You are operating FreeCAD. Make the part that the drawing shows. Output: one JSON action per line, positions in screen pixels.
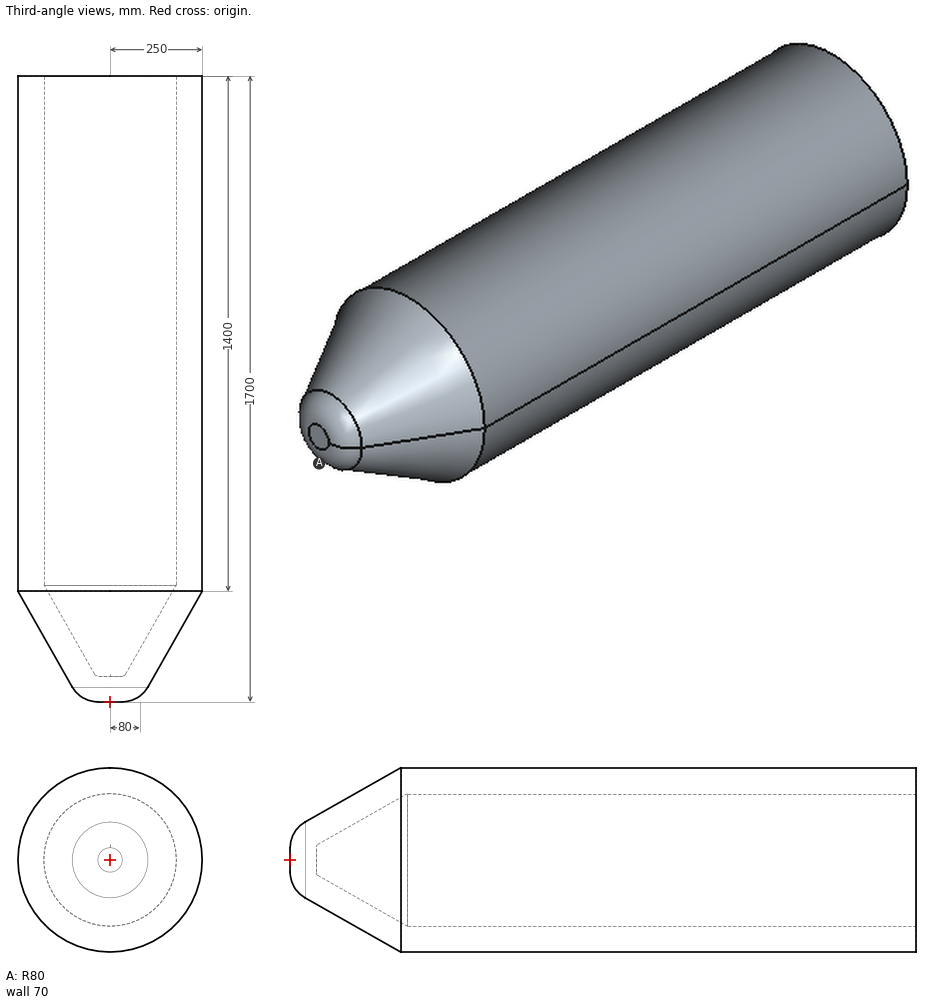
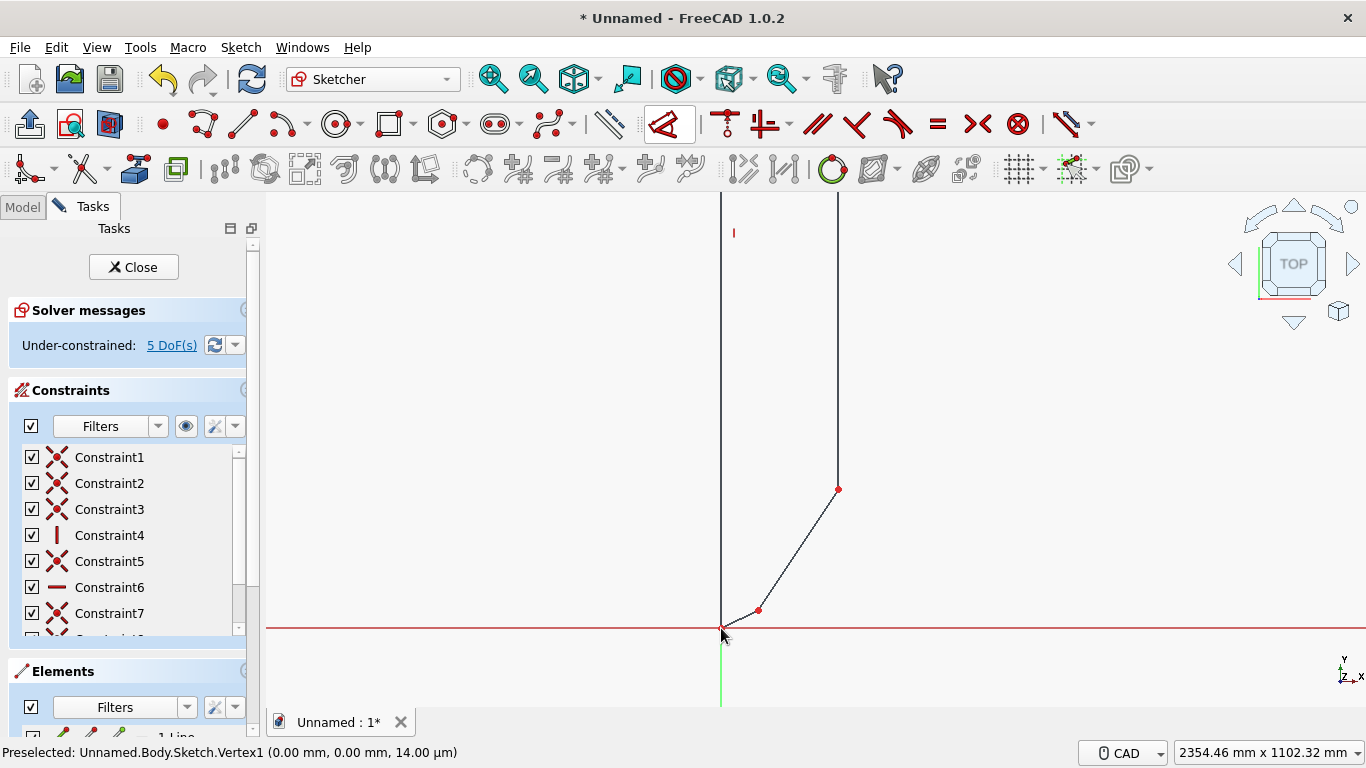
{"action": "left_click", "coordinate": [747, 616]}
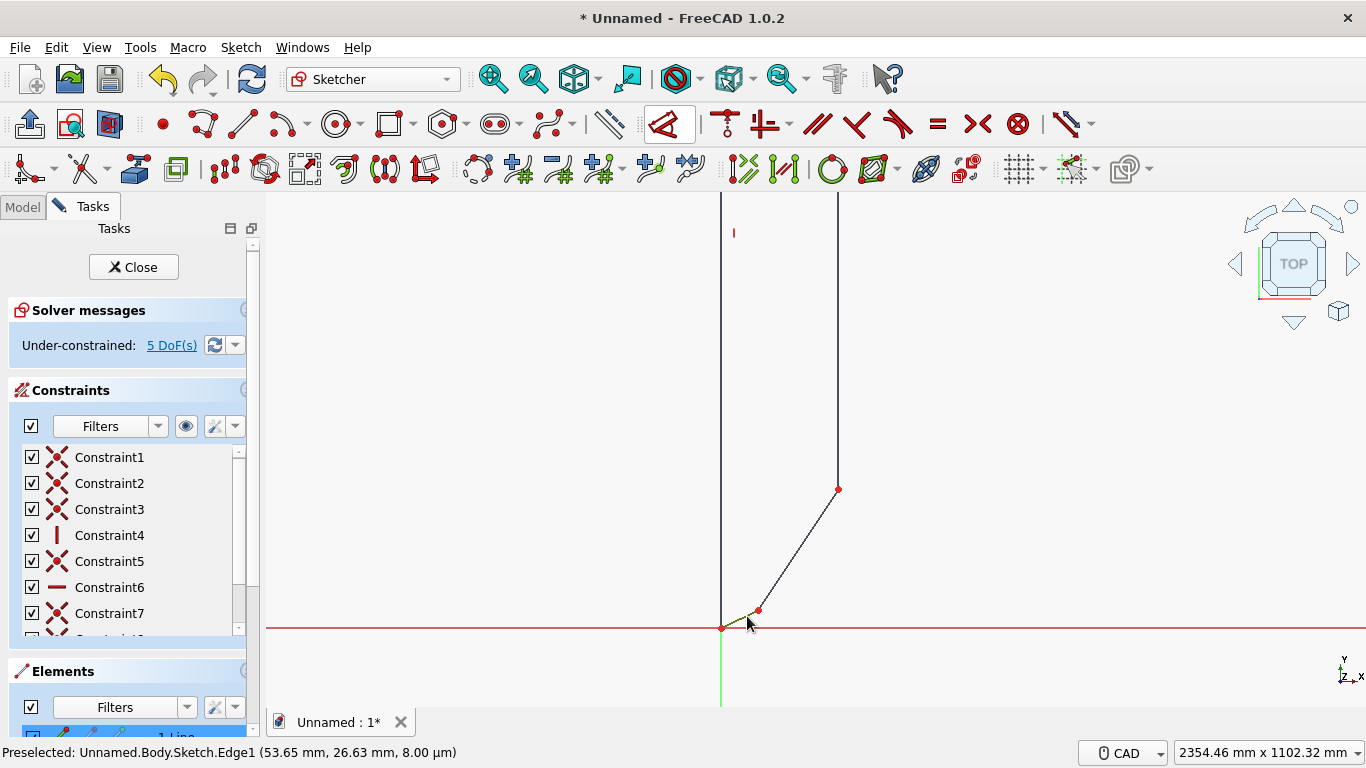
{"action": "key", "text": "h"}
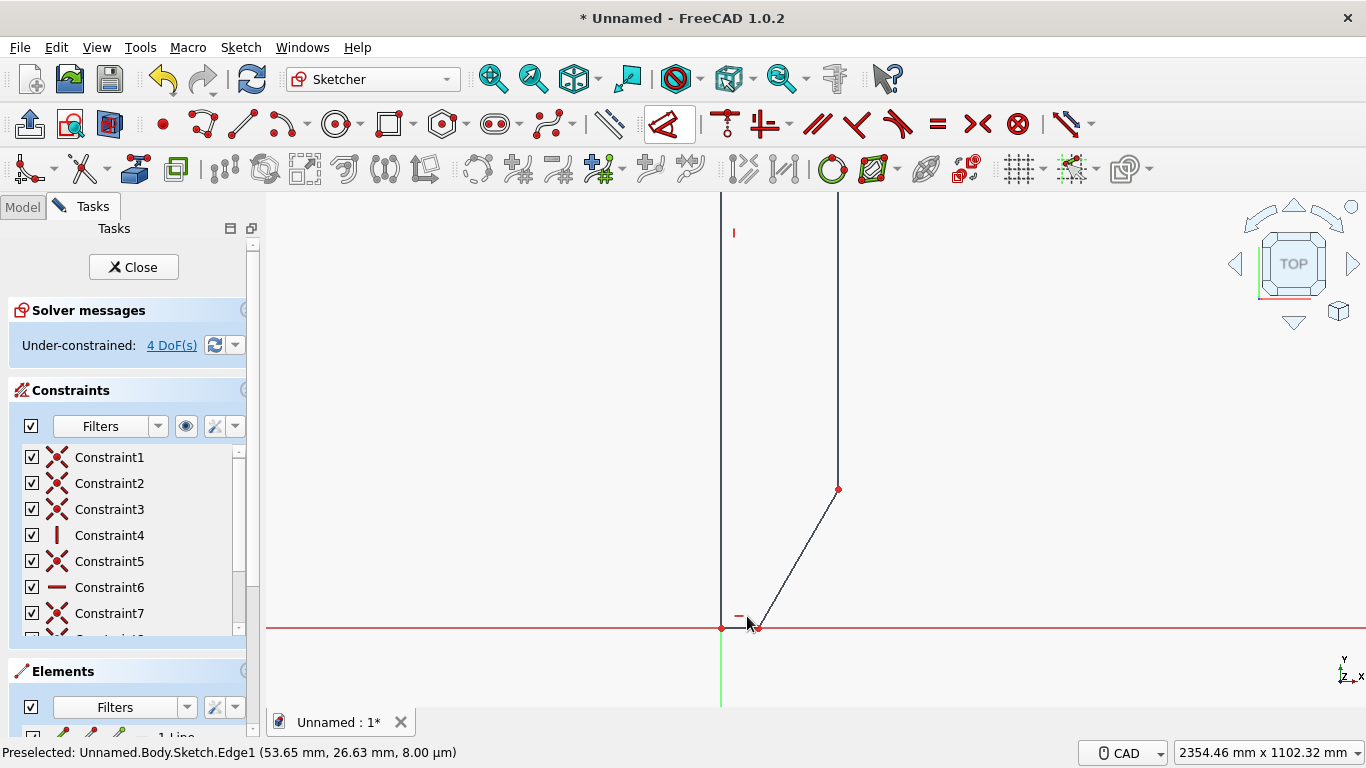
{"action": "scroll", "coordinate": [733, 628], "scroll_direction": "up", "scroll_amount": 2}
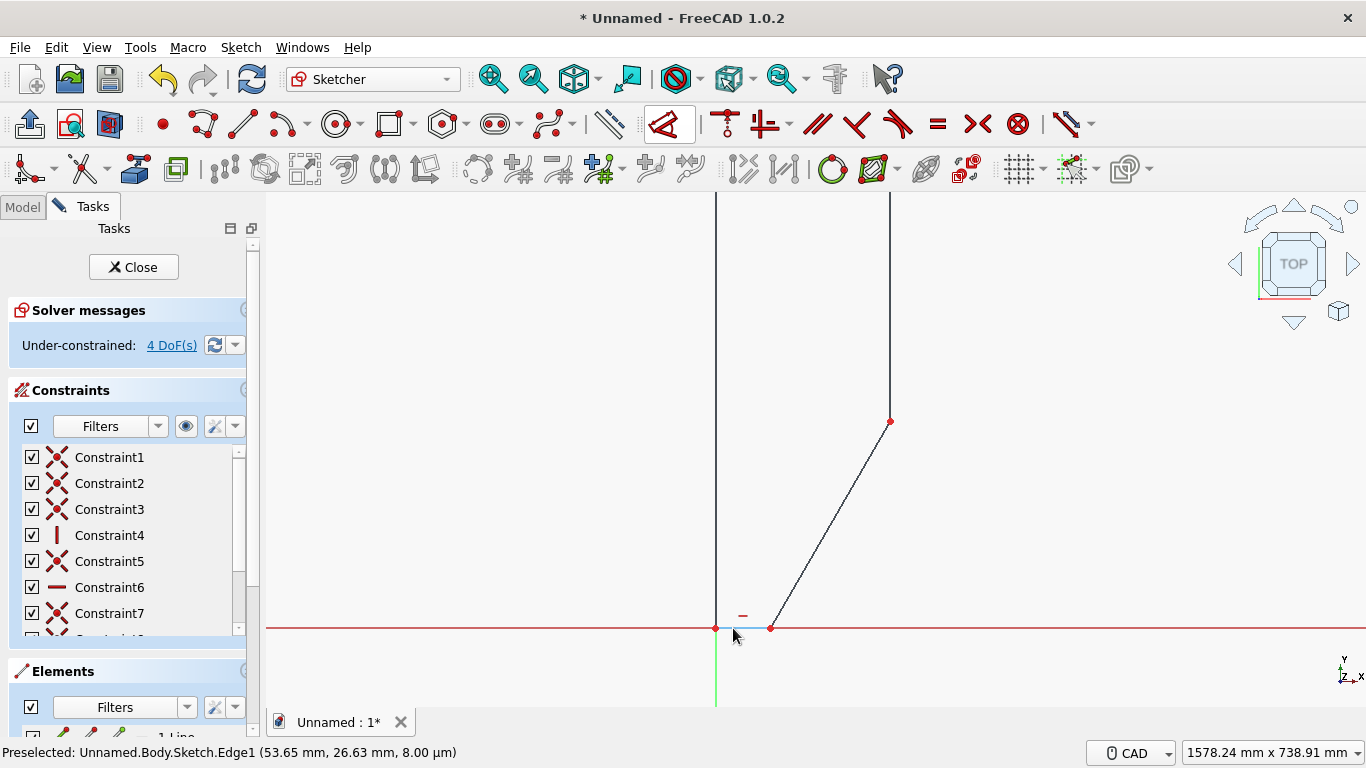
{"action": "left_click", "coordinate": [732, 628]}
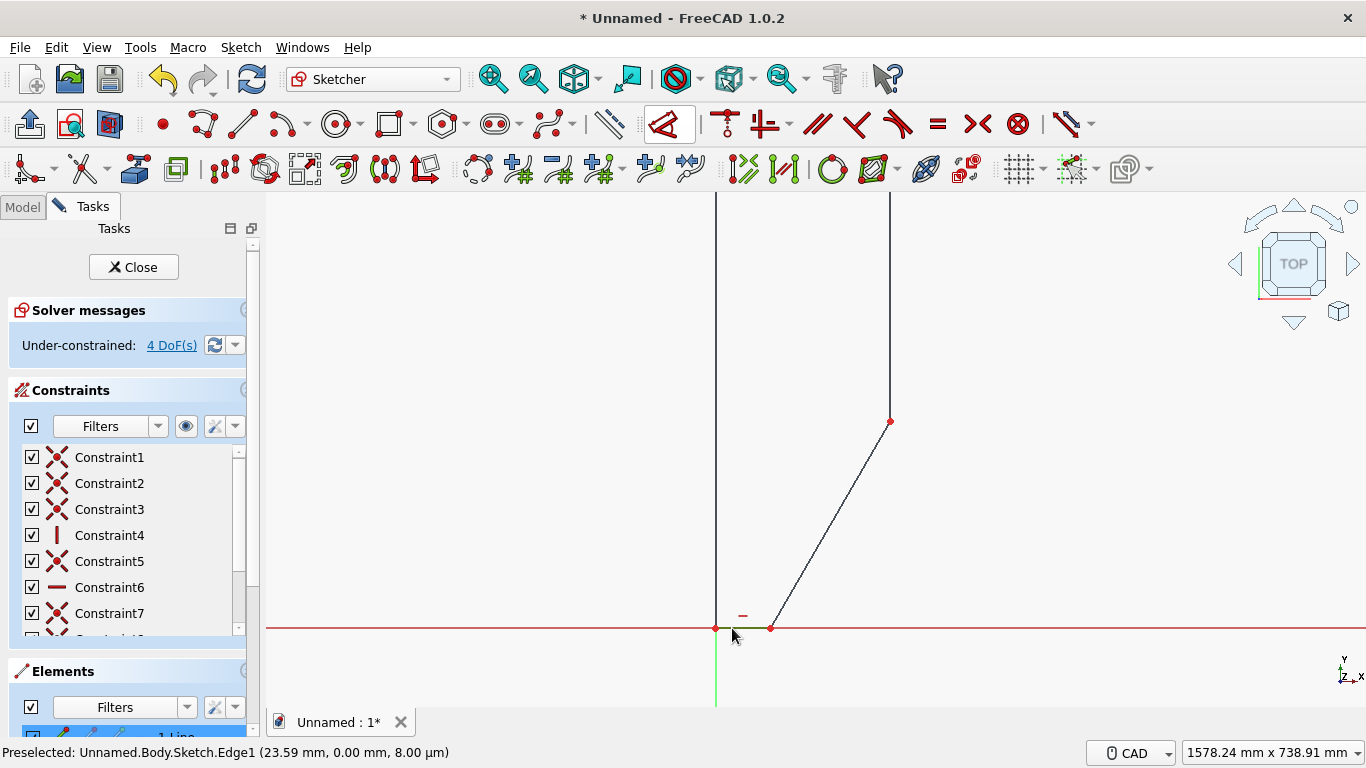
{"action": "left_click", "coordinate": [690, 124]}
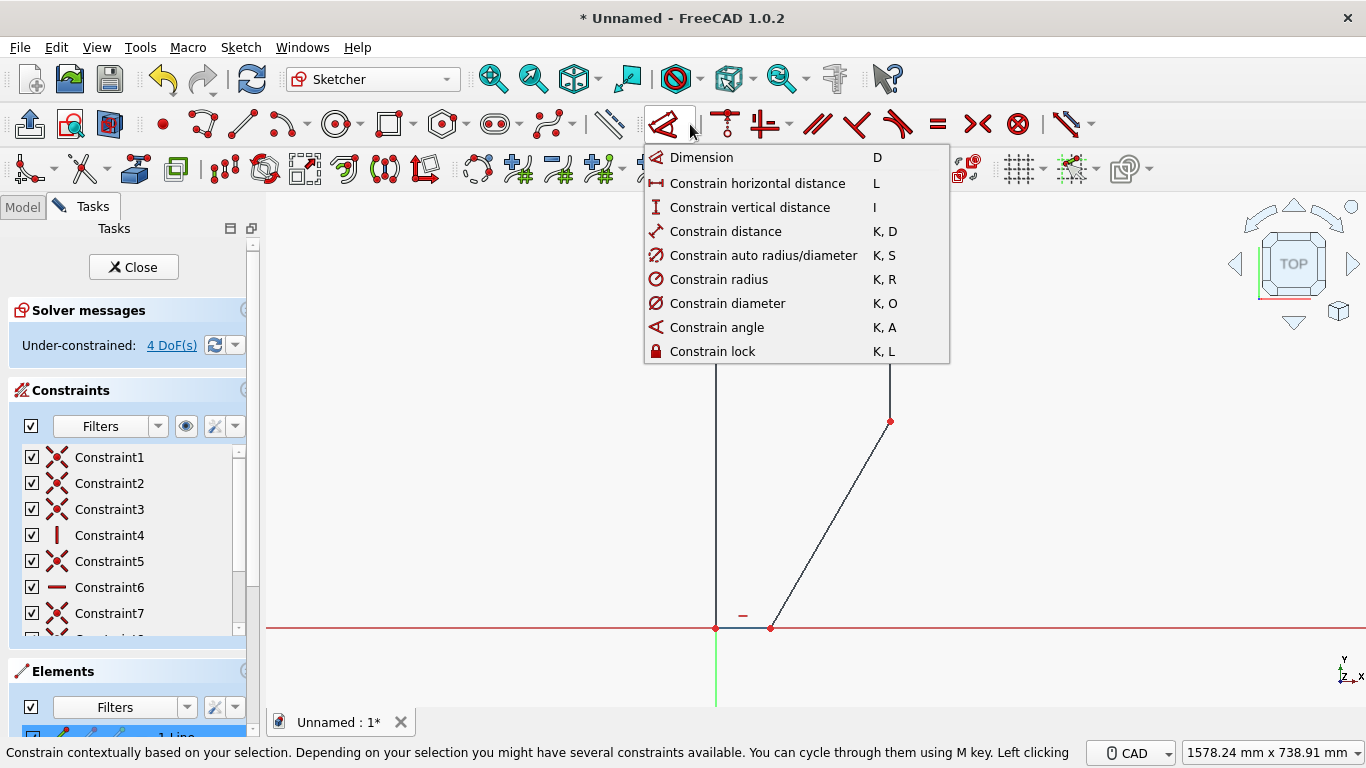
{"action": "left_click", "coordinate": [797, 183]}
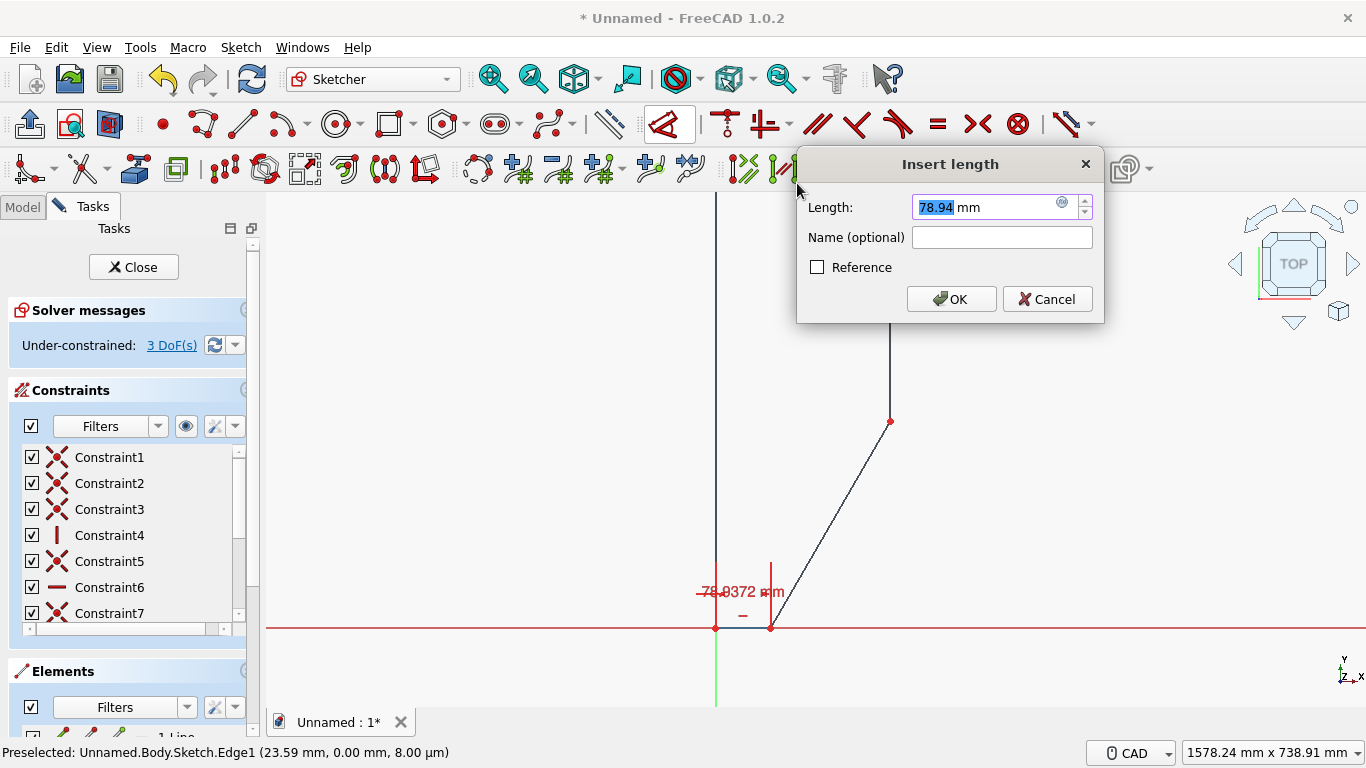
{"action": "type", "text": "80"}
{"action": "key", "text": "Return"}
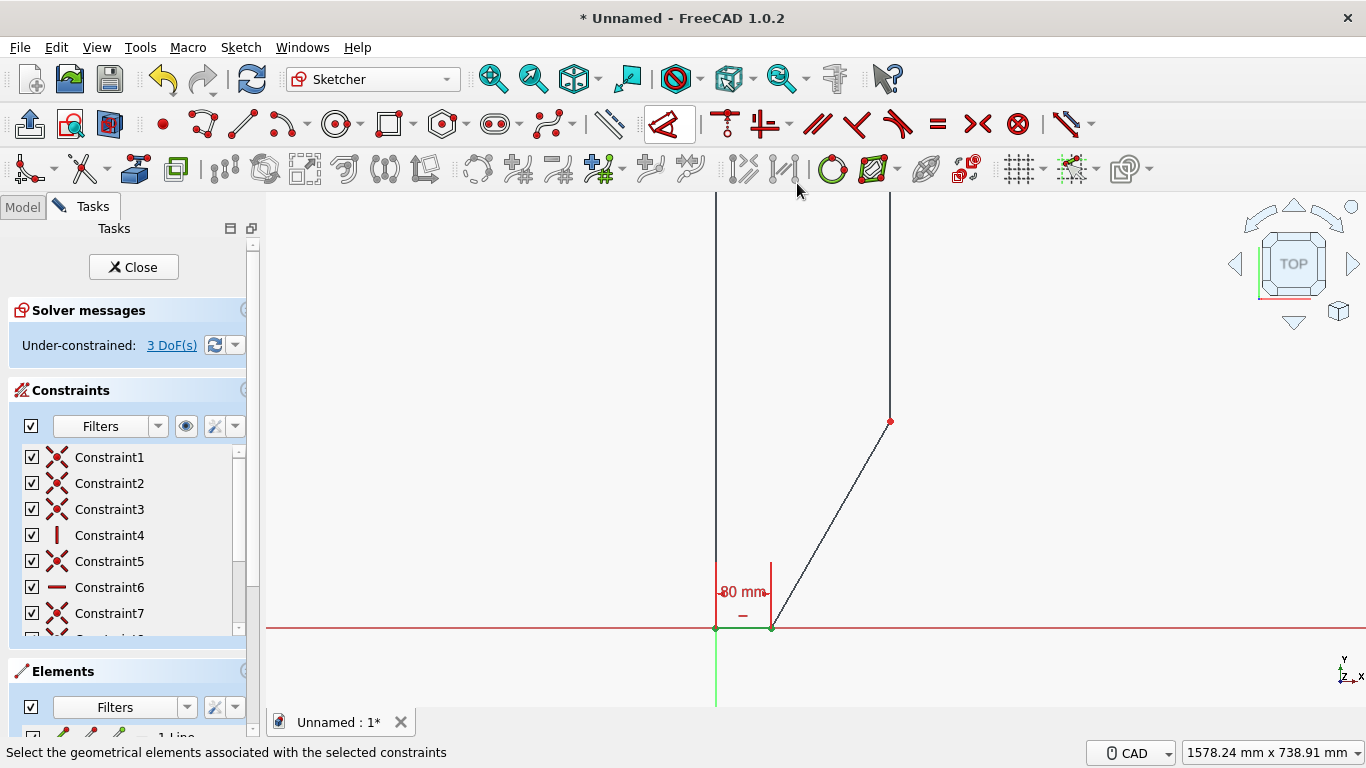
{"action": "scroll", "coordinate": [724, 628], "scroll_direction": "down", "scroll_amount": 6}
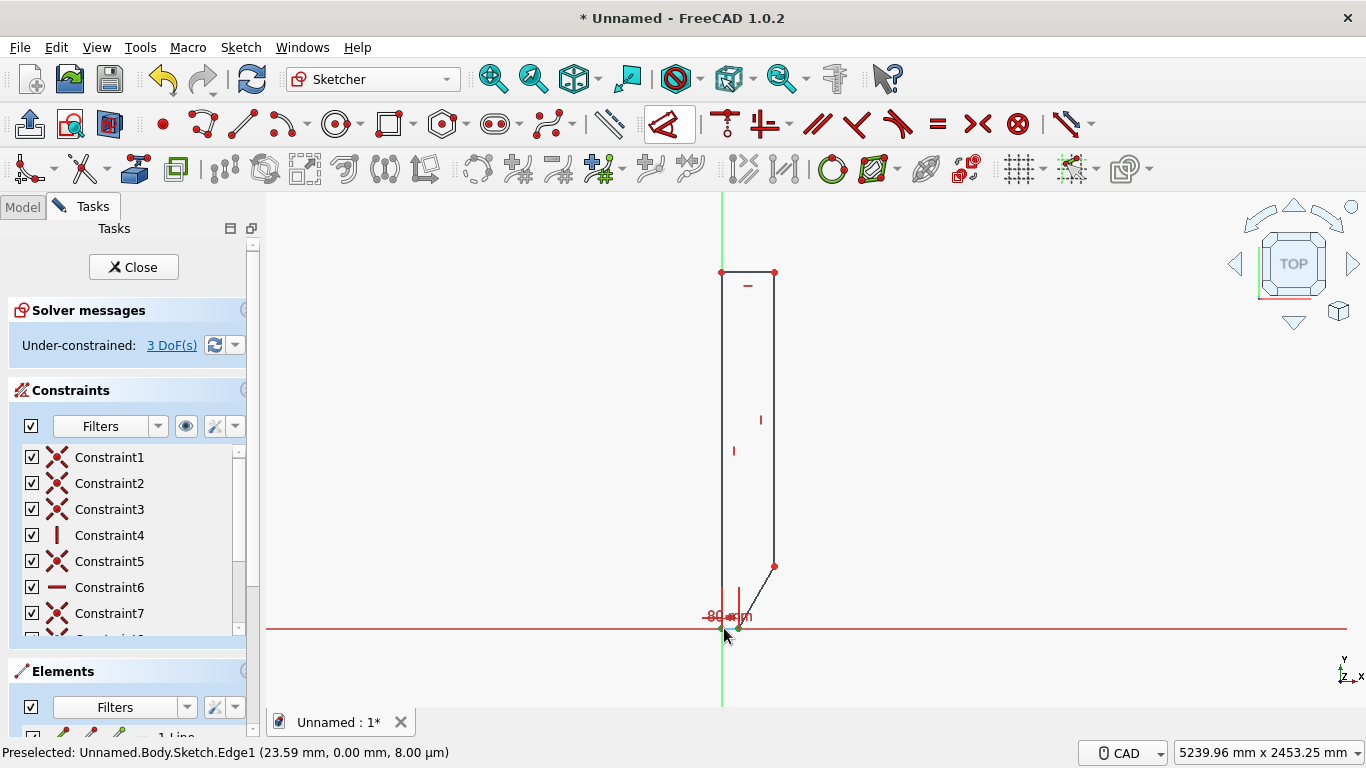
{"action": "left_click", "coordinate": [759, 272]}